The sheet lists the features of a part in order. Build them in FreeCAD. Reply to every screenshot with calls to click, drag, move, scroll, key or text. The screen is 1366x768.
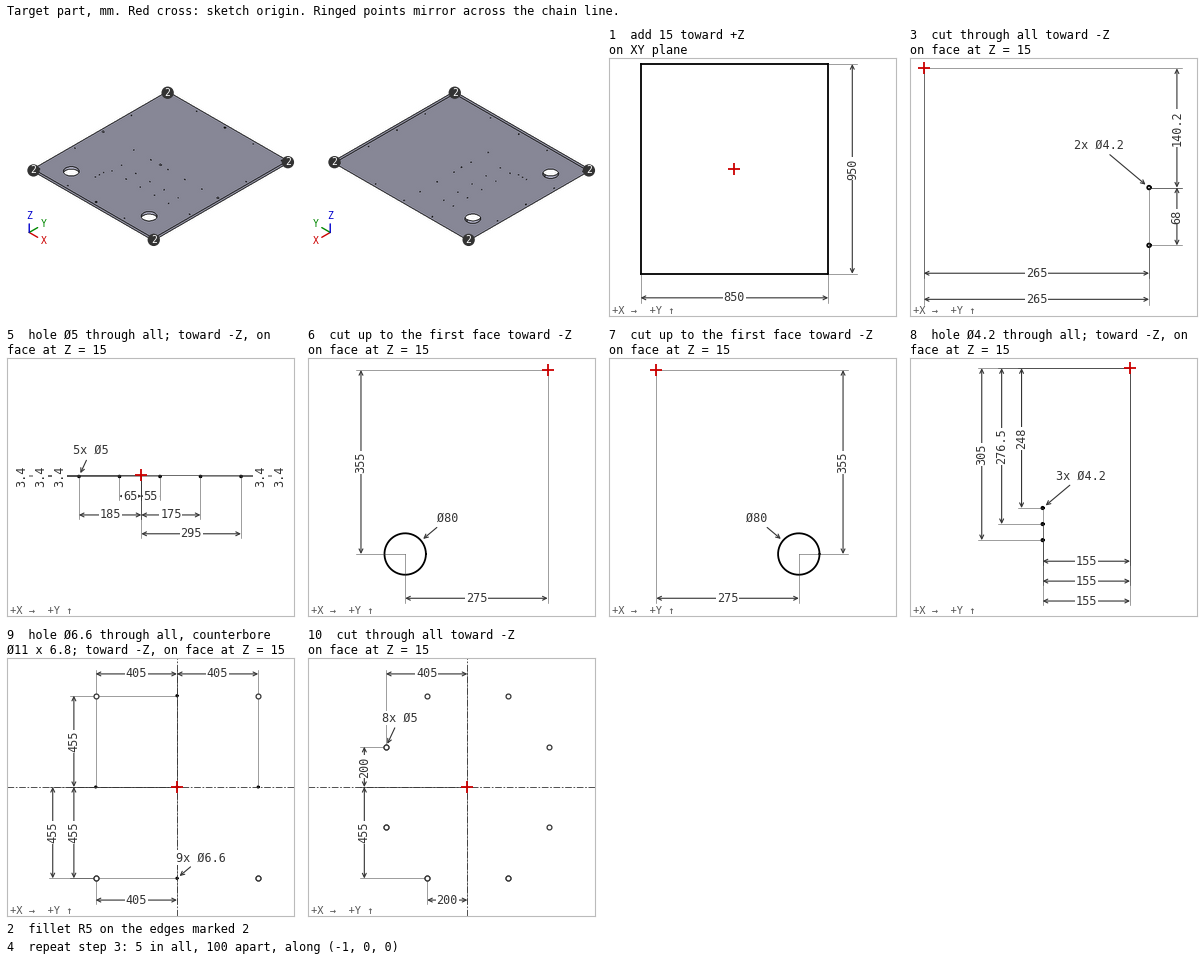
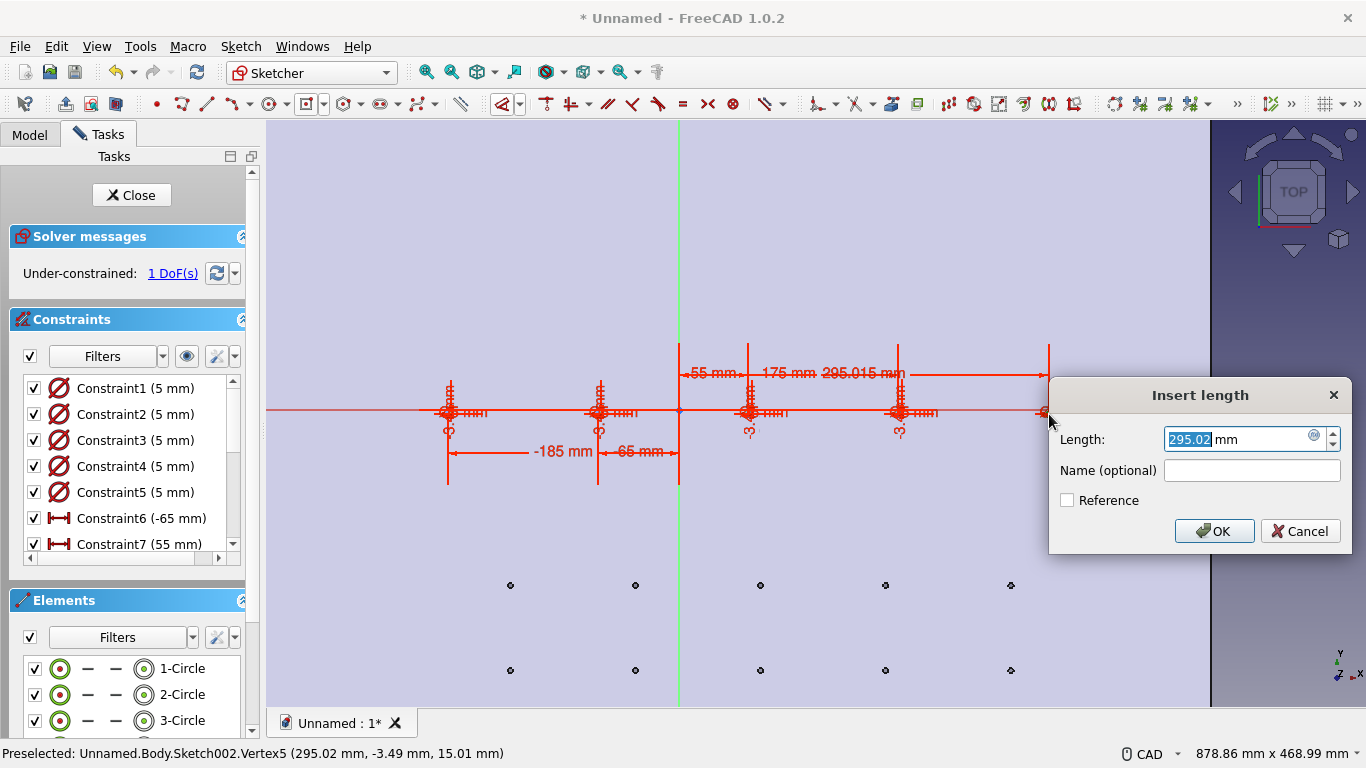
text(295)
key(Return)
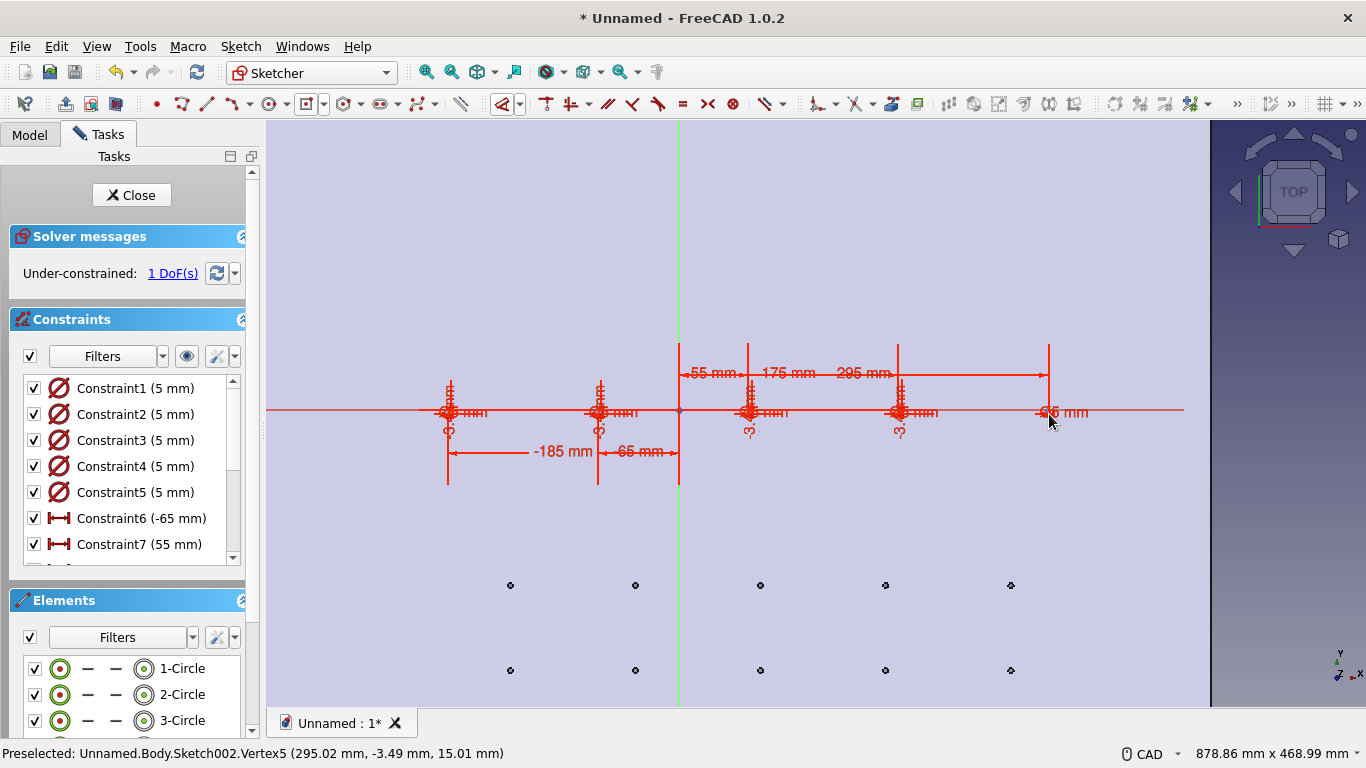
scroll(1049, 414, up, 12)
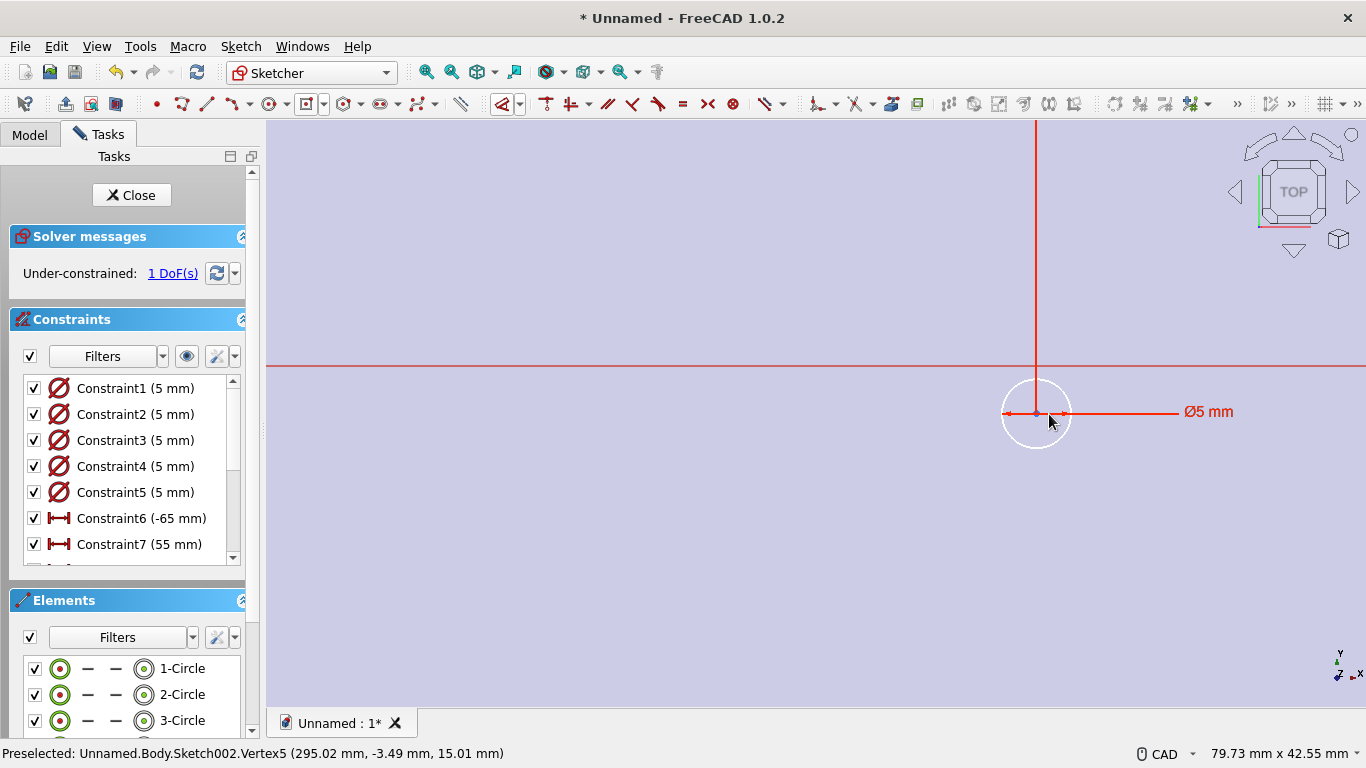
click(1036, 414)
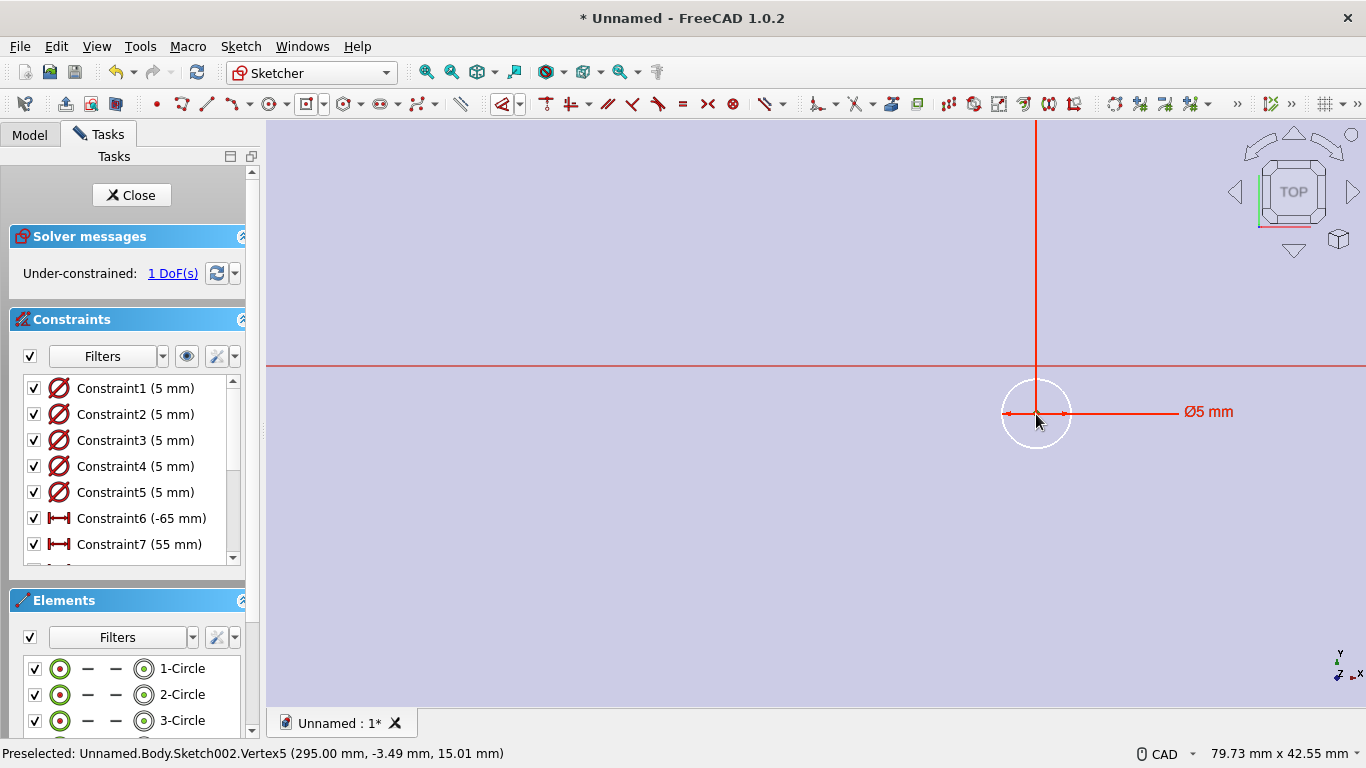
key(i)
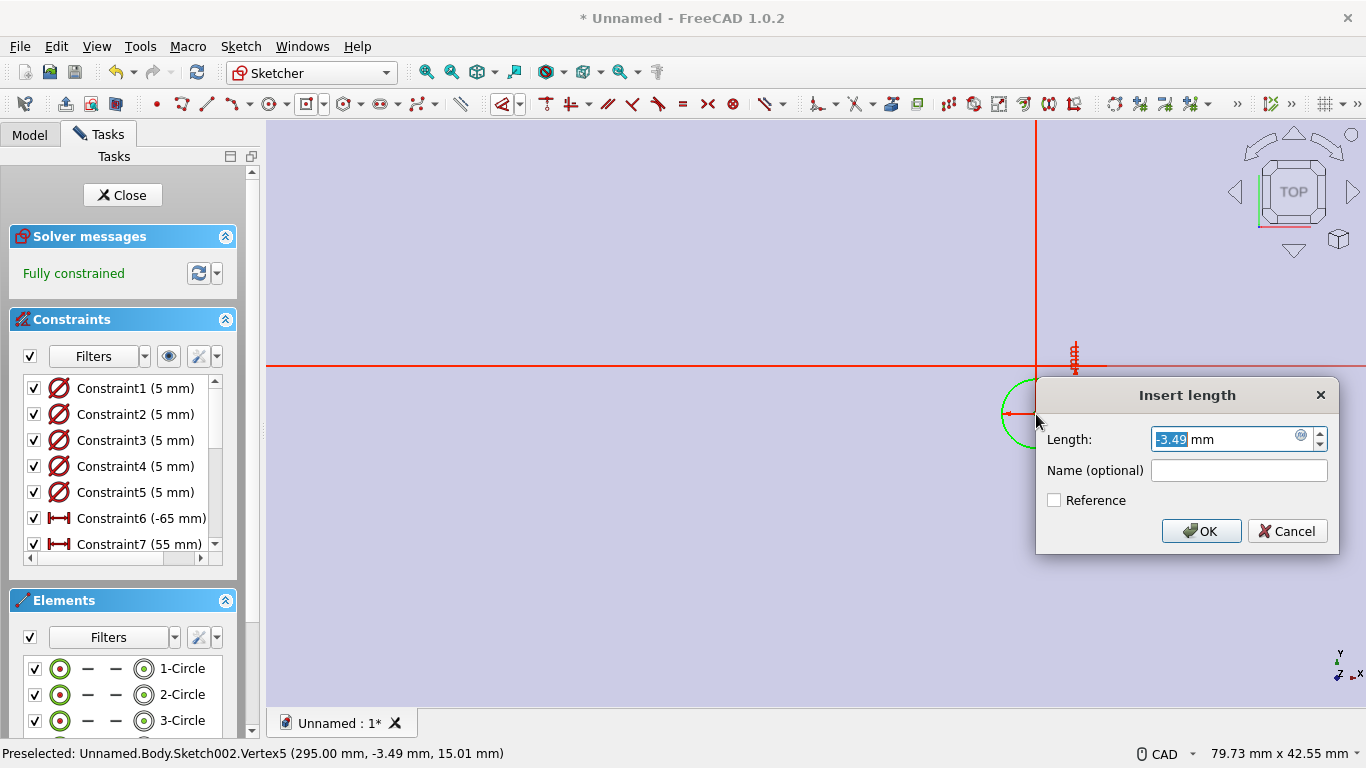
text(-3.4)
key(Return)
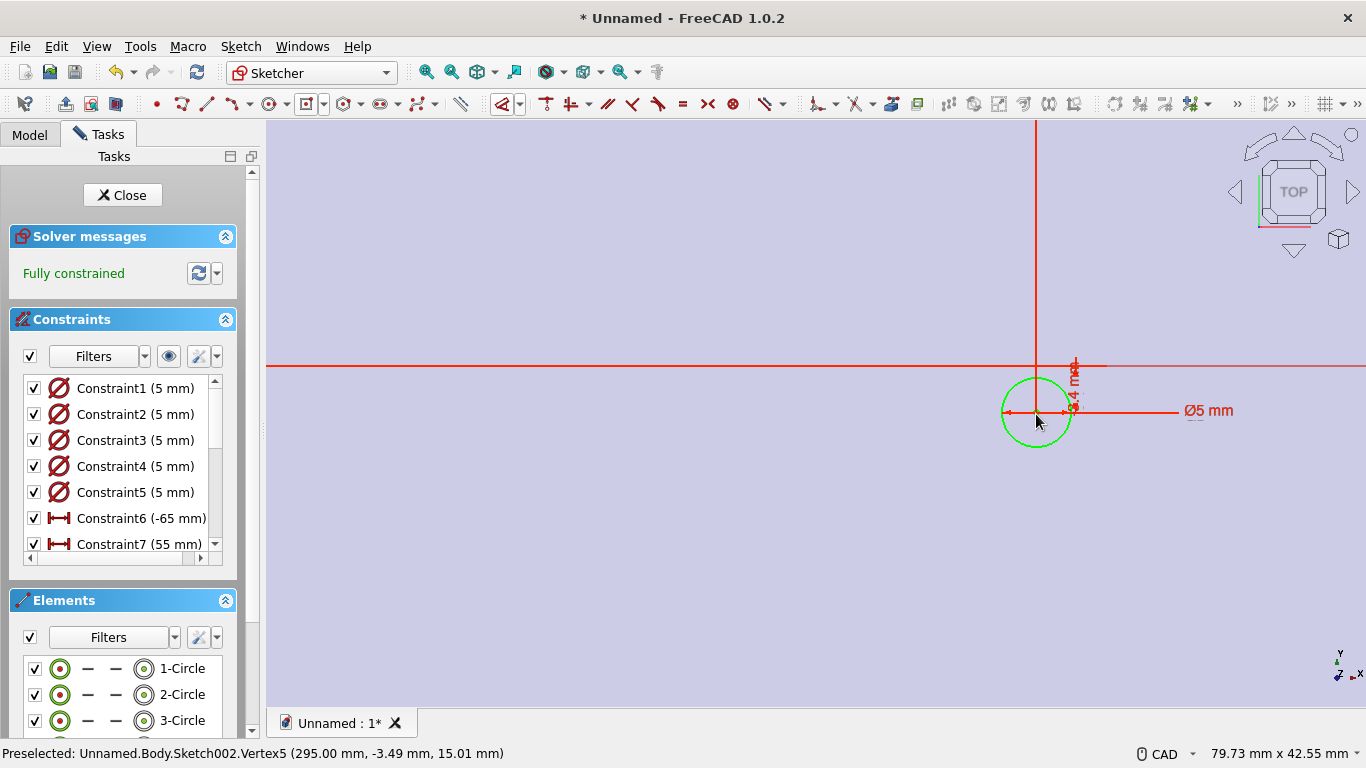
click(123, 195)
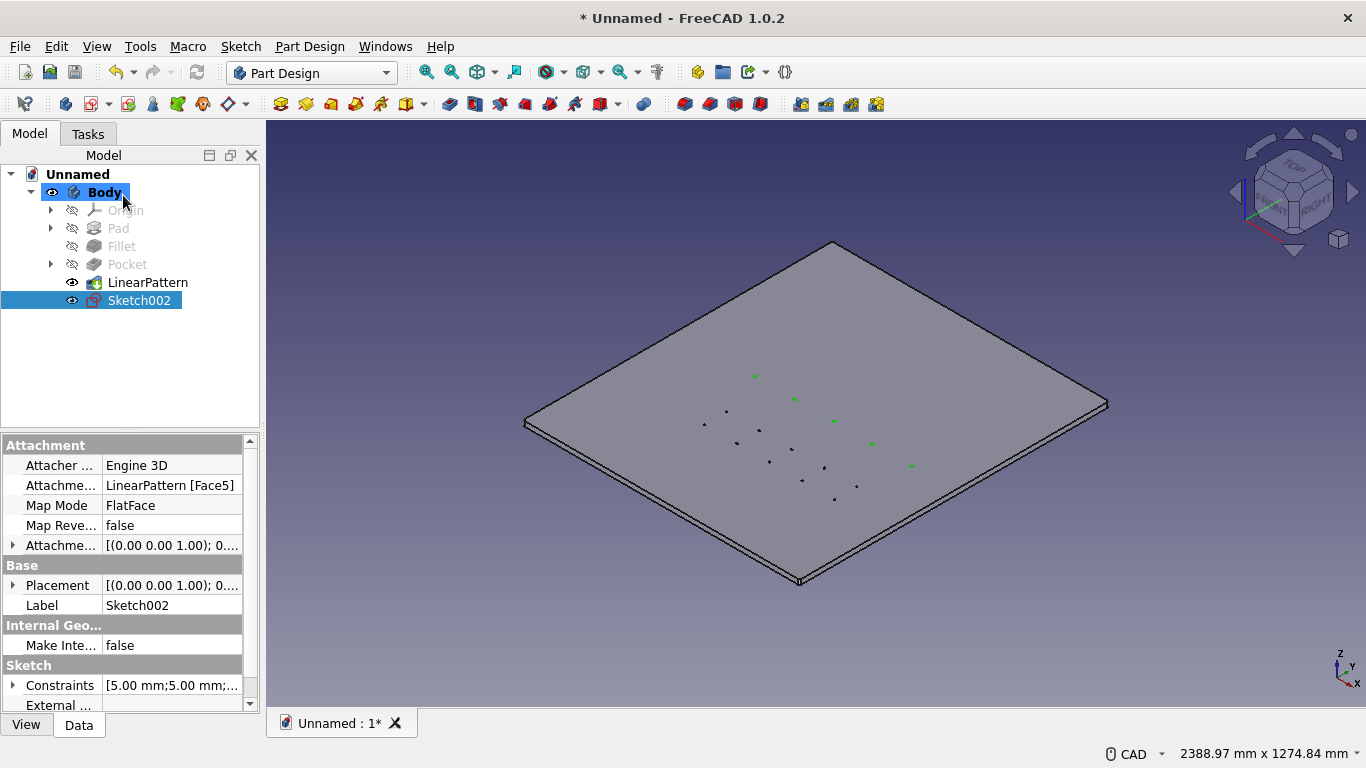
click(475, 104)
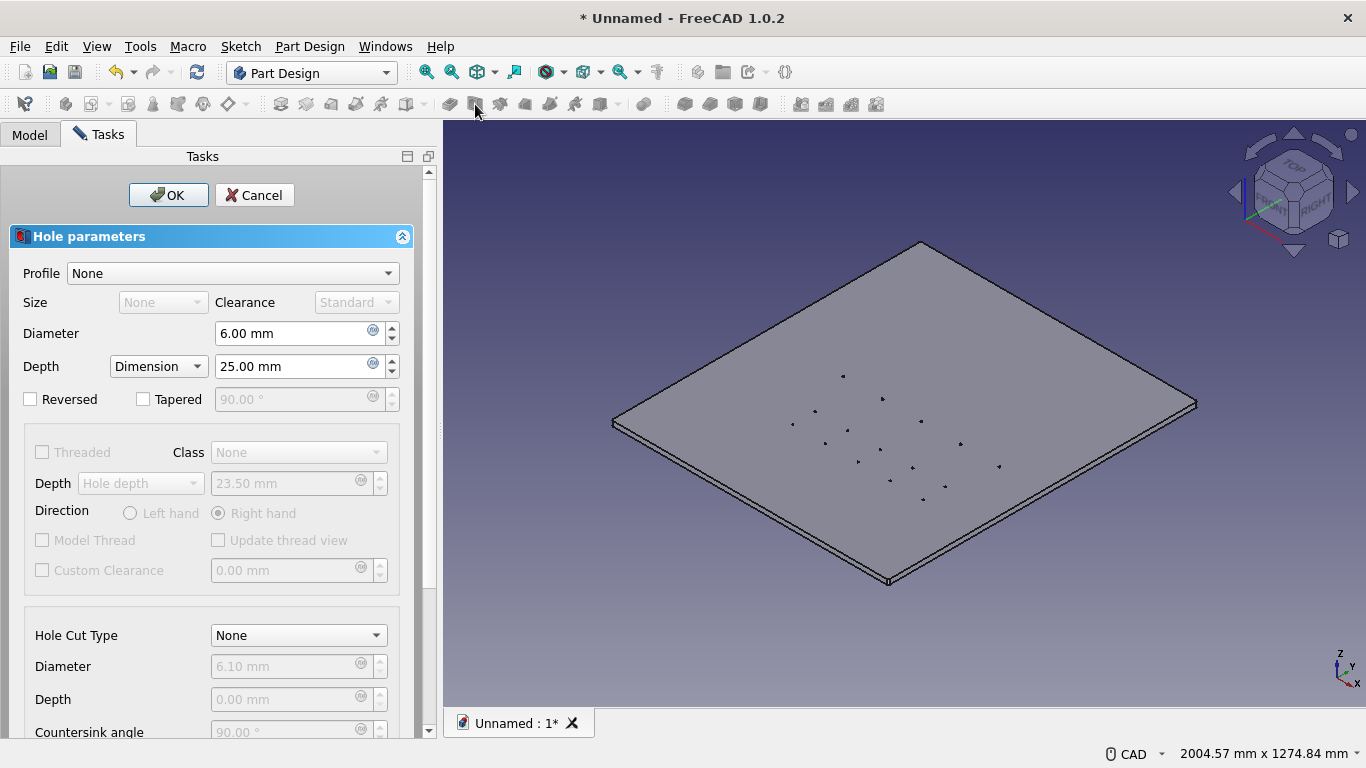
triple_click(300, 334)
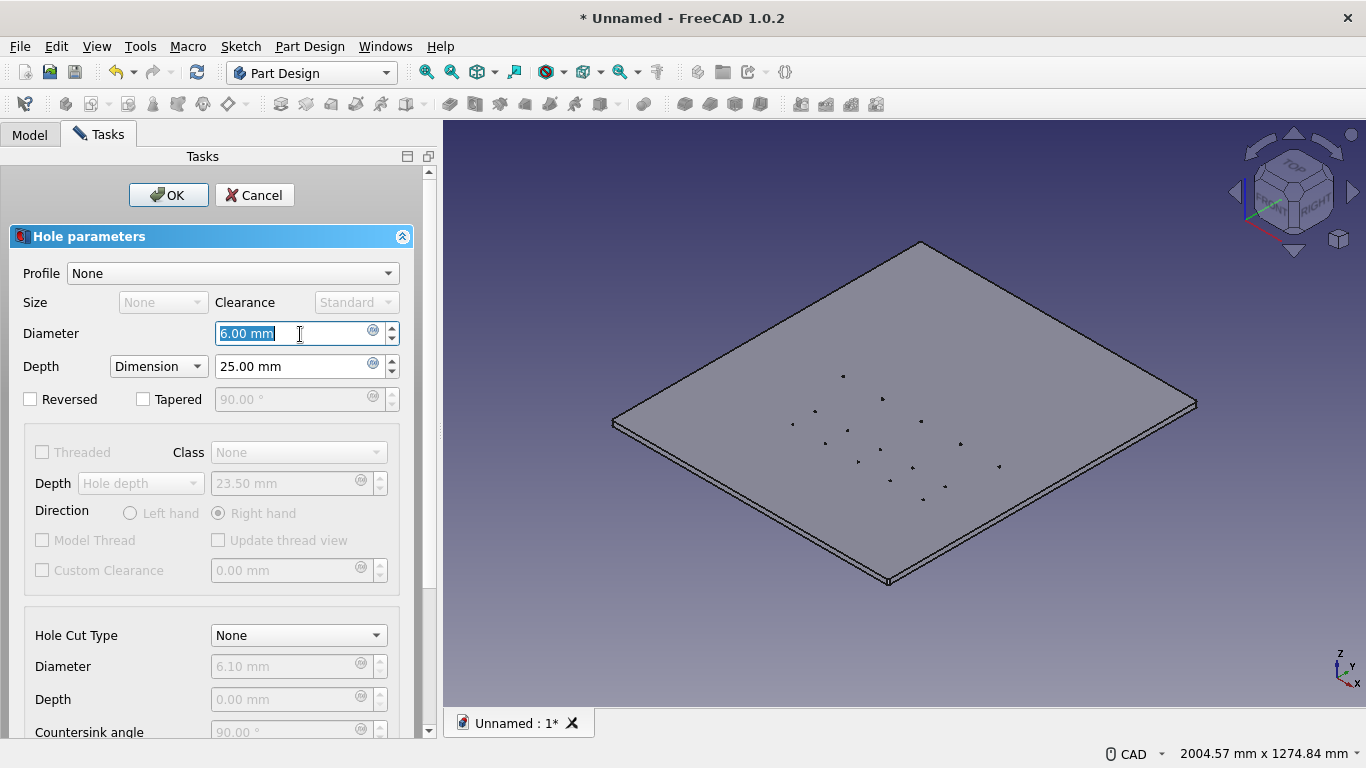
text(5)
key(Tab)